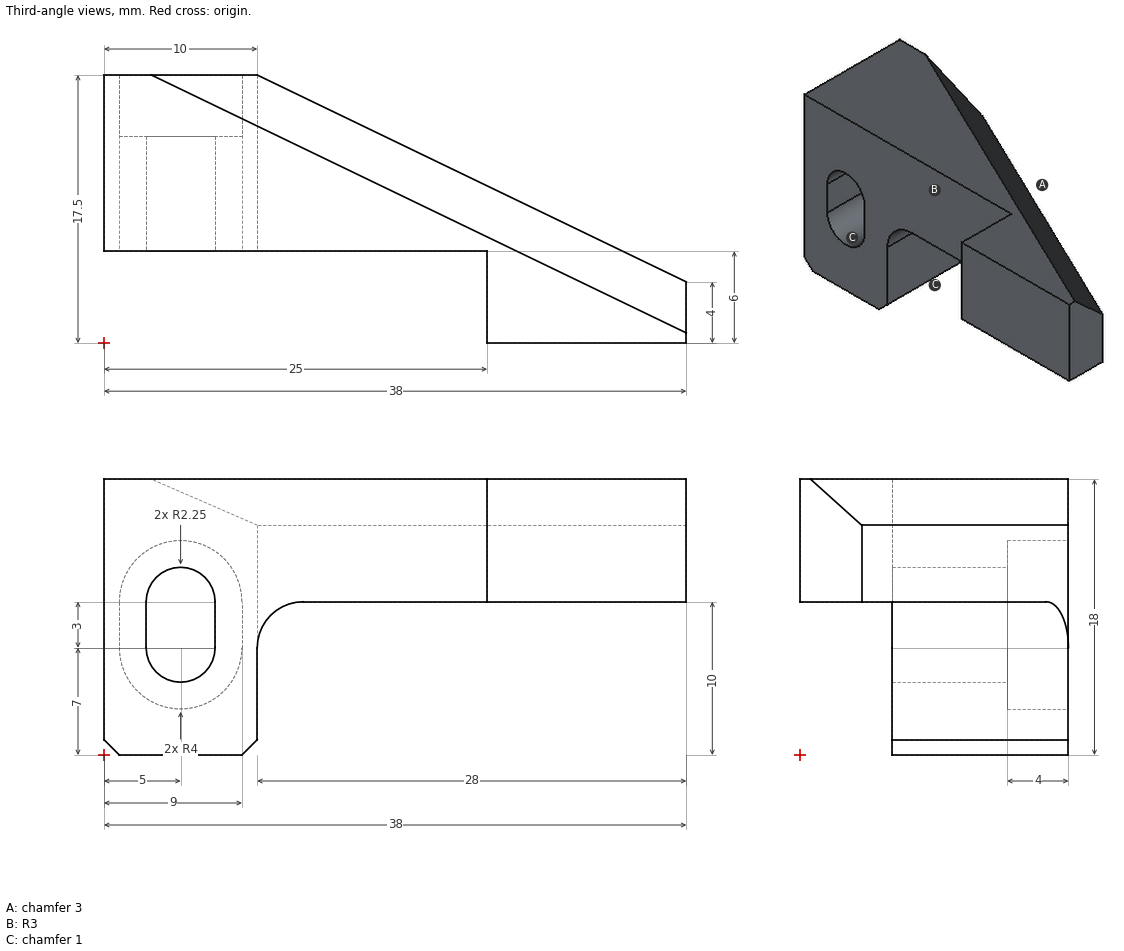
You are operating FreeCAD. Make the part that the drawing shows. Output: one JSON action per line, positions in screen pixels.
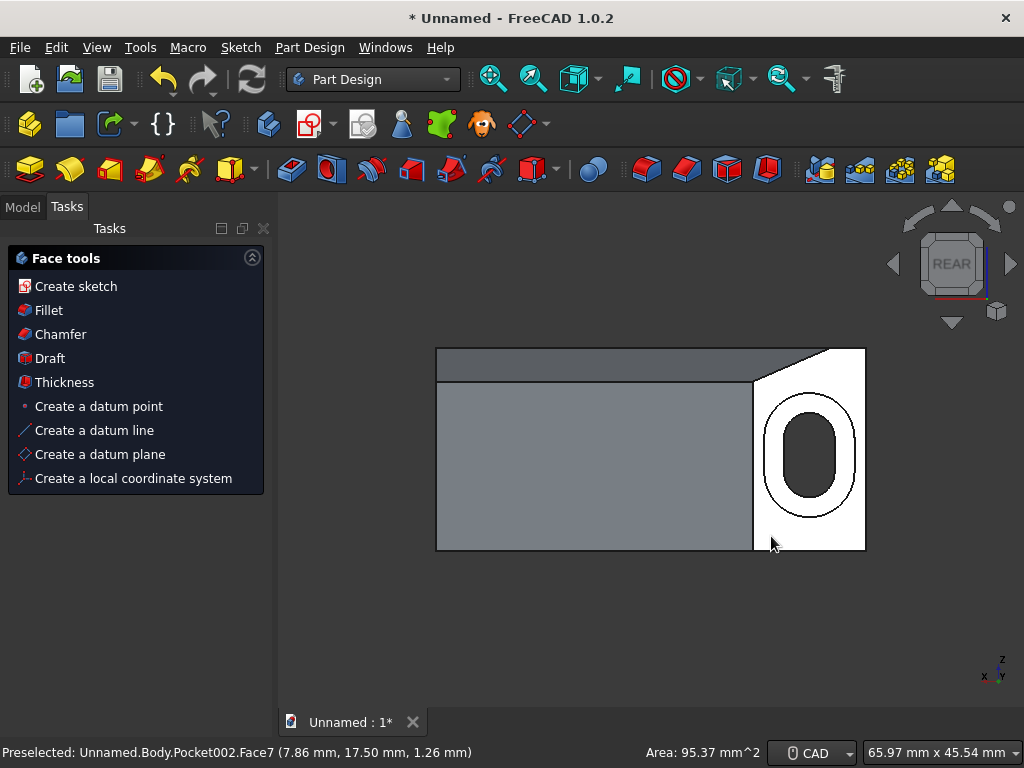
{"action": "left_click", "coordinate": [310, 124]}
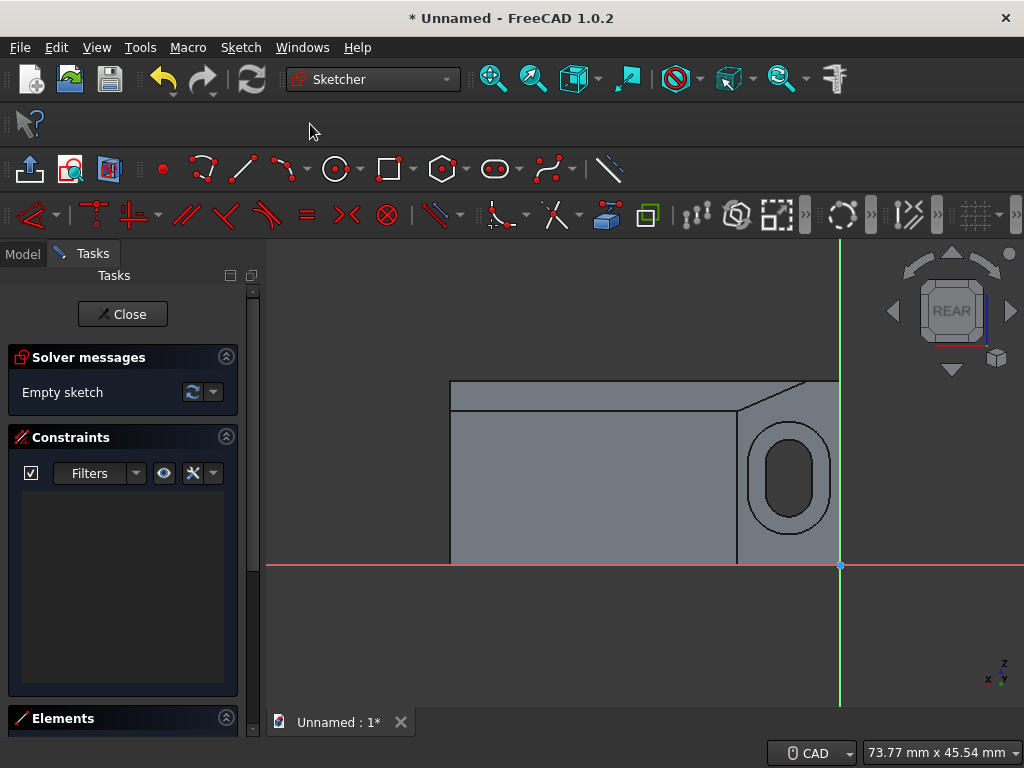
{"action": "scroll", "coordinate": [294, 287], "scroll_direction": "down", "scroll_amount": 1}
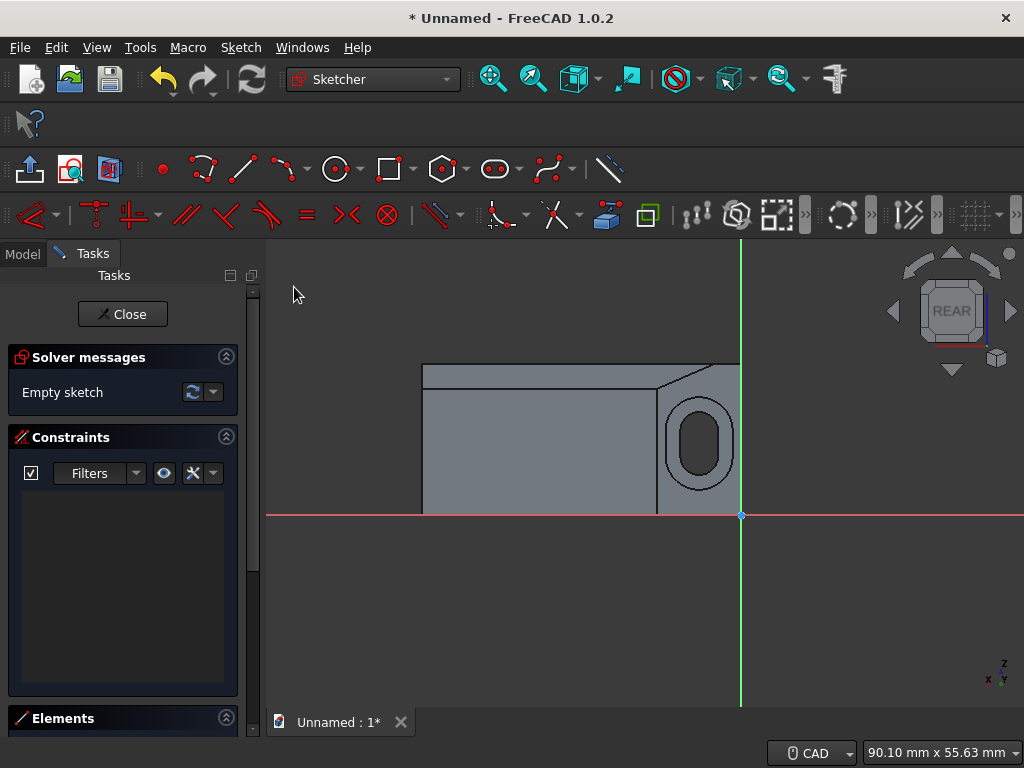
{"action": "key", "text": "g r"}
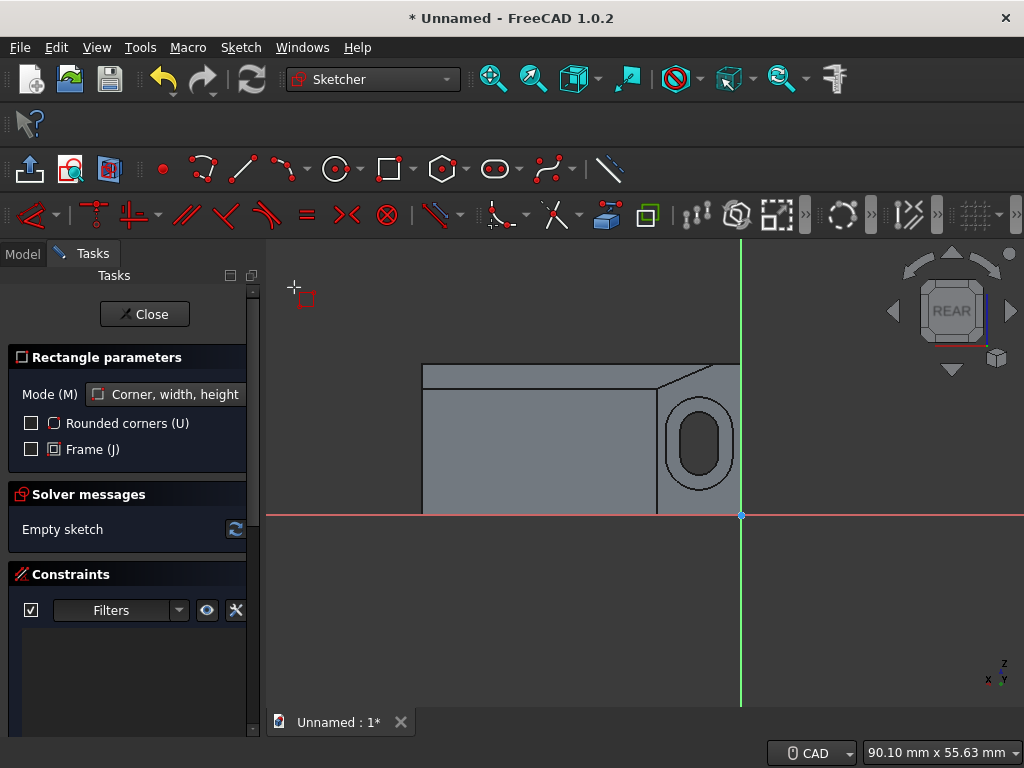
{"action": "left_click", "coordinate": [422, 431]}
{"action": "left_click", "coordinate": [657, 515]}
{"action": "key", "text": "Escape"}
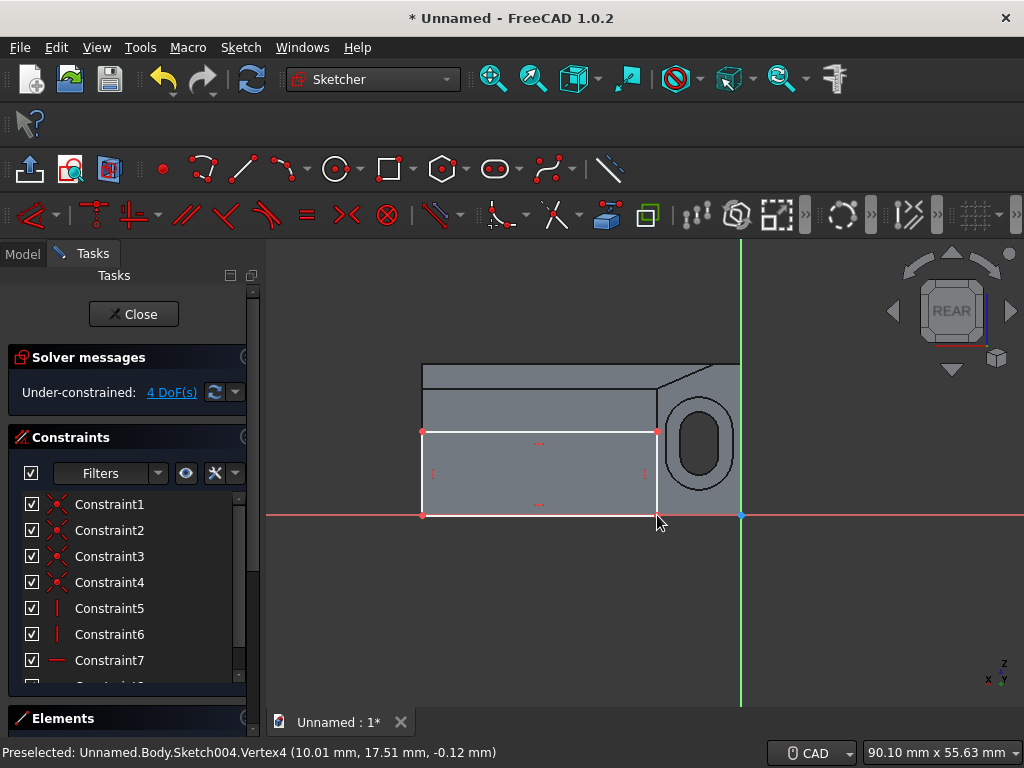
{"action": "left_click", "coordinate": [422, 516]}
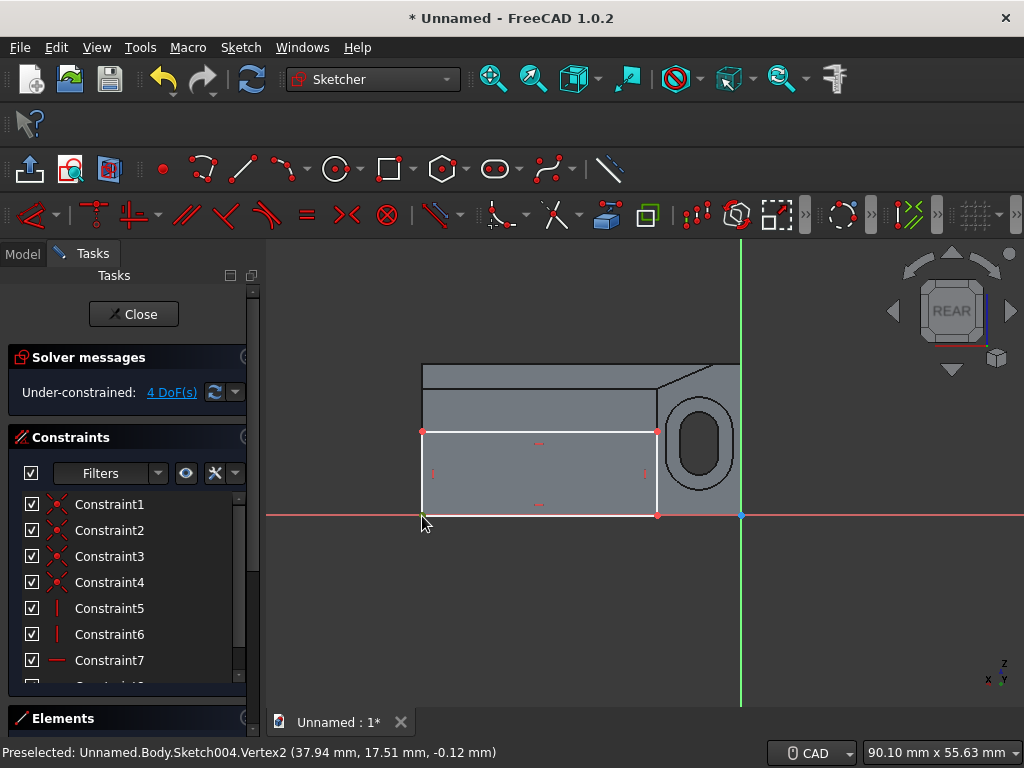
{"action": "left_click", "coordinate": [334, 515]}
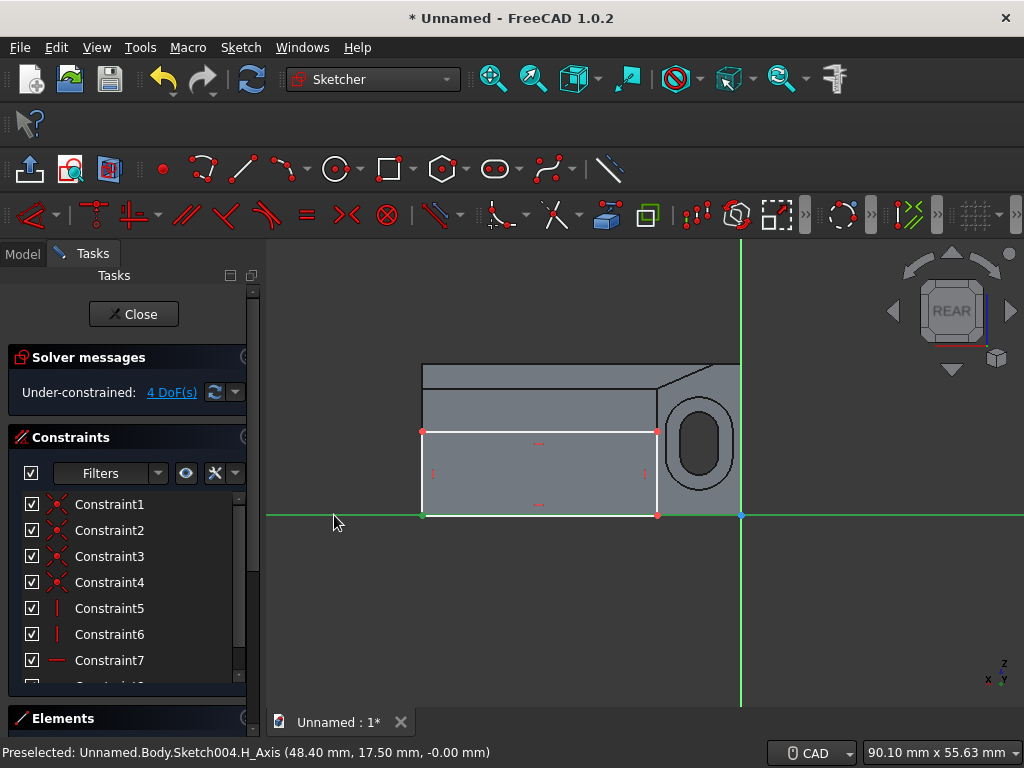
{"action": "key", "text": "c"}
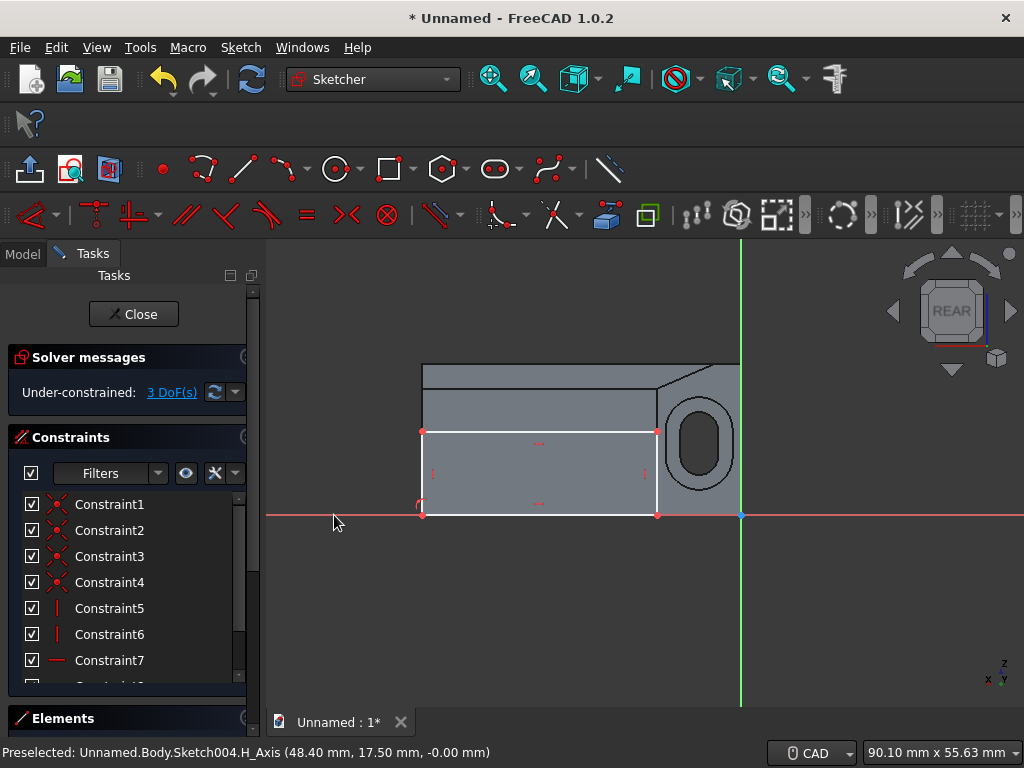
{"action": "key", "text": "d"}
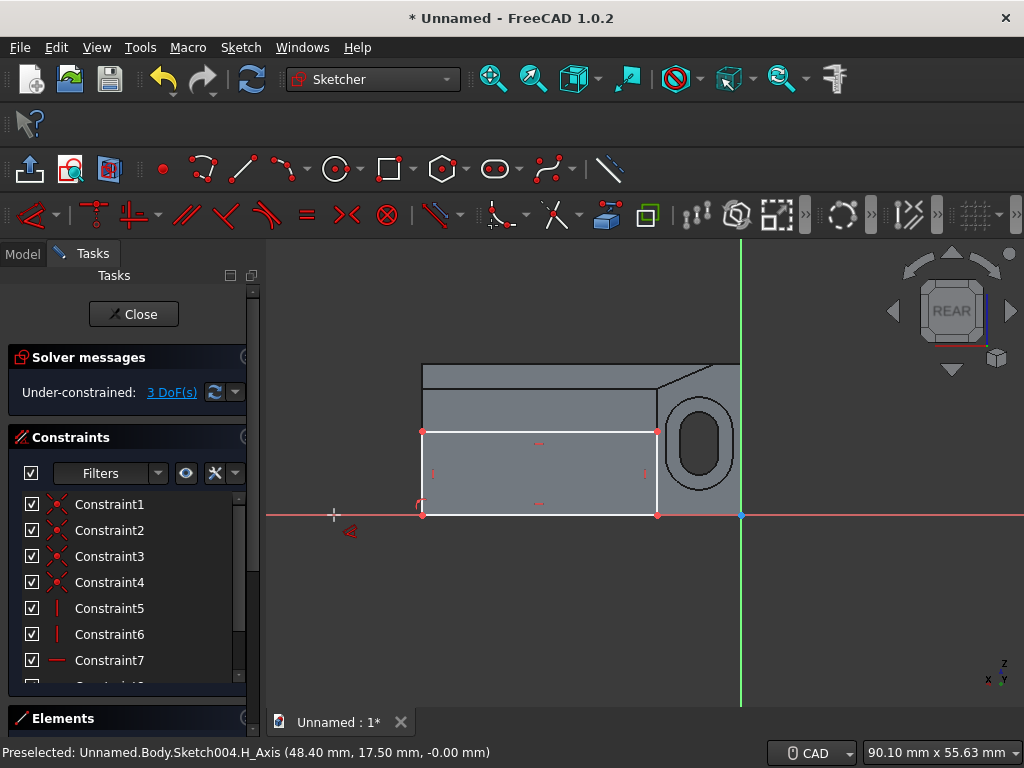
{"action": "left_click", "coordinate": [422, 457]}
{"action": "left_click", "coordinate": [388, 474]}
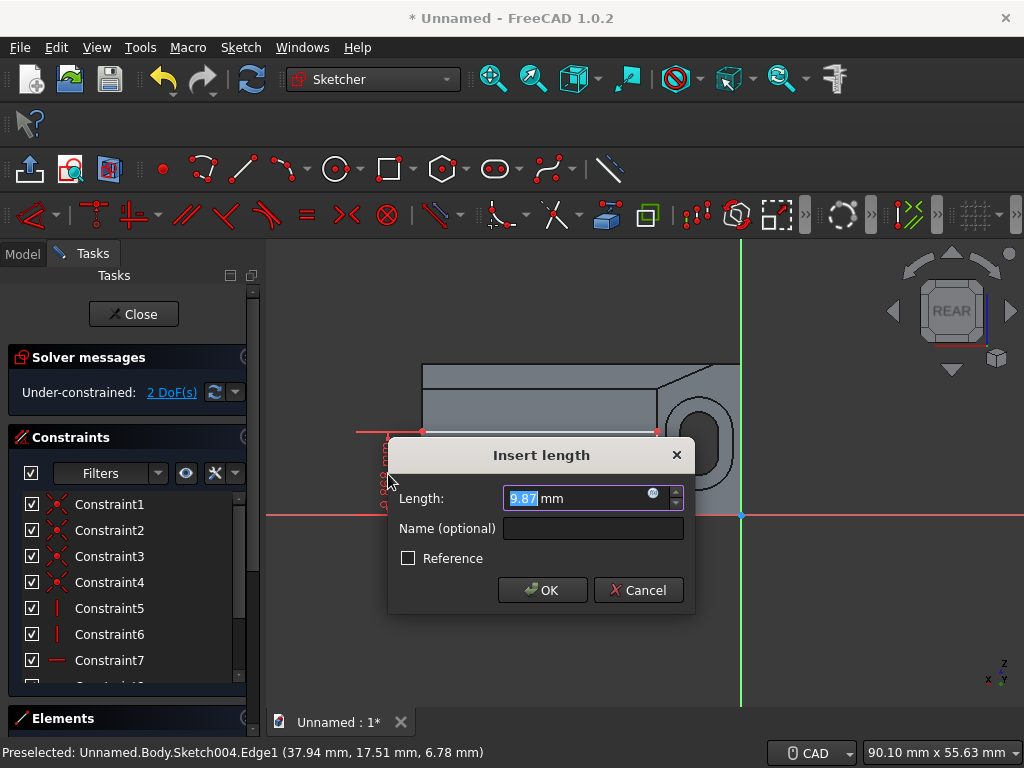
{"action": "type", "text": "10"}
{"action": "key", "text": "Return"}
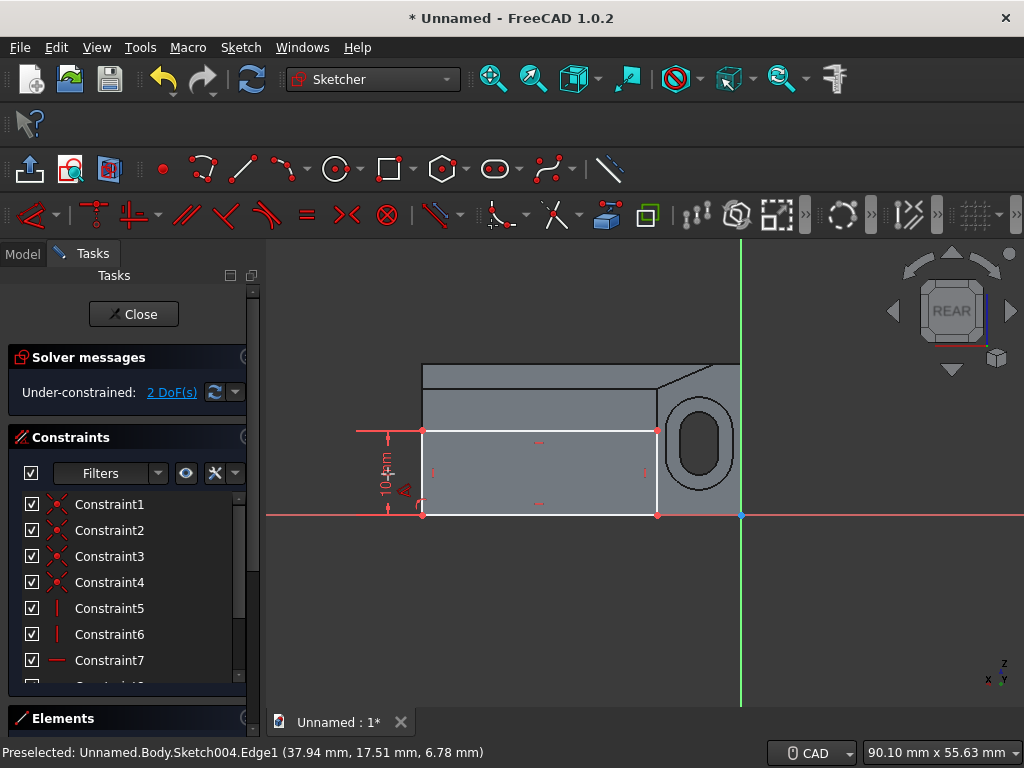
{"action": "left_click", "coordinate": [492, 515]}
{"action": "left_click", "coordinate": [539, 549]}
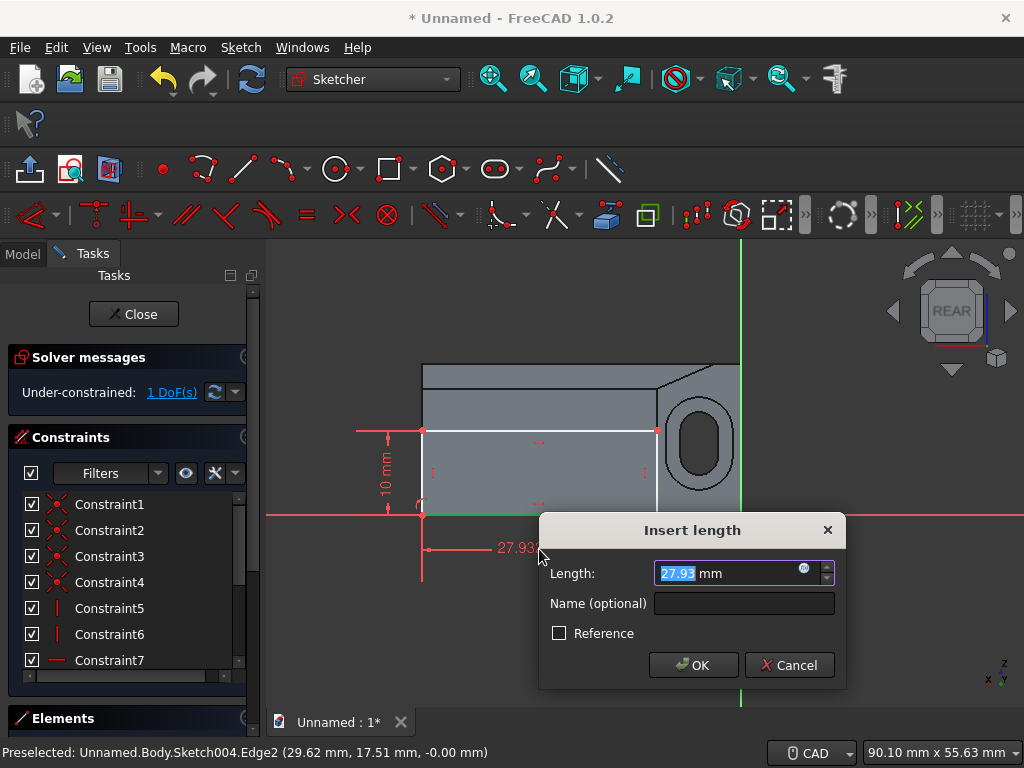
{"action": "type", "text": "28"}
{"action": "key", "text": "Return"}